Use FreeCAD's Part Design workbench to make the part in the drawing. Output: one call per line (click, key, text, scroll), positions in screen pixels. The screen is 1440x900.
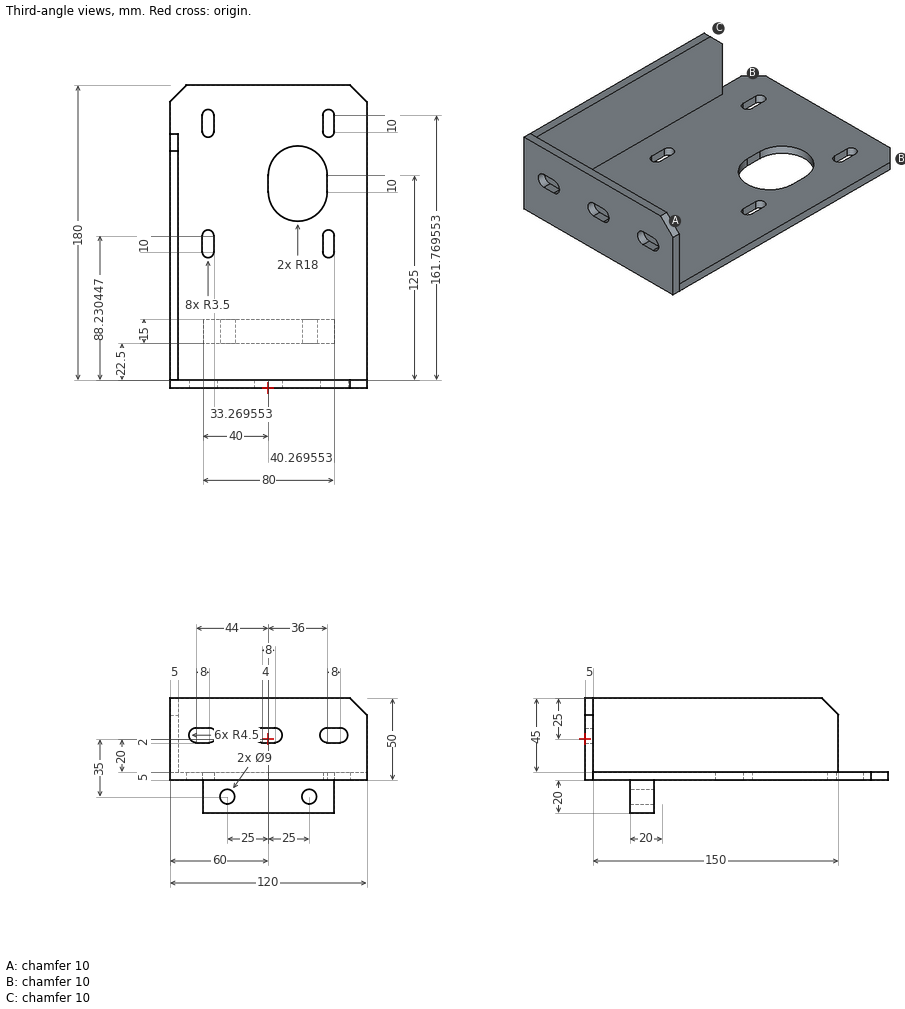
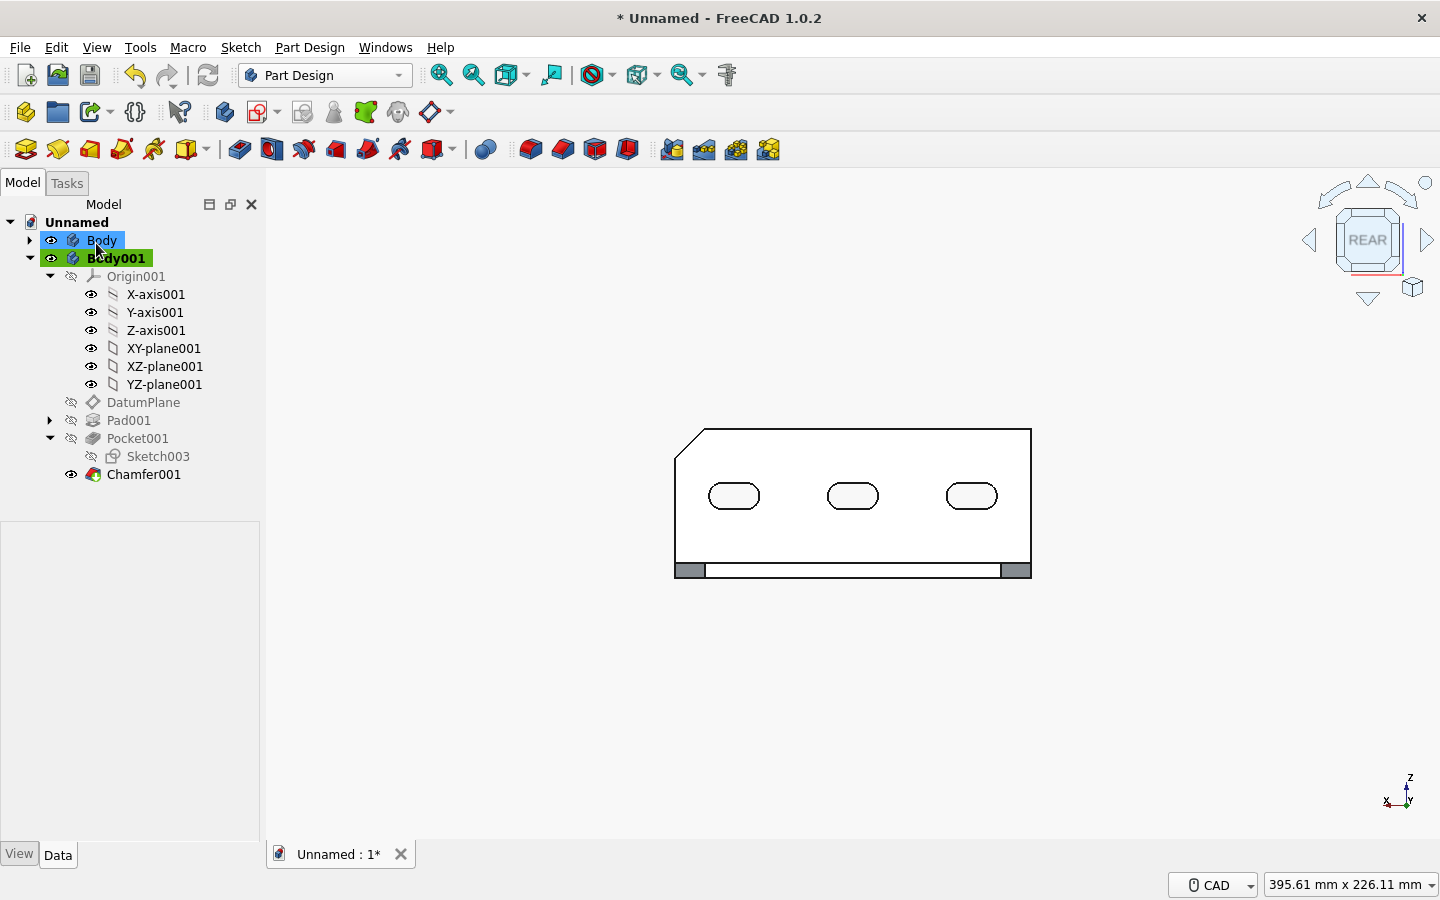
click(442, 76)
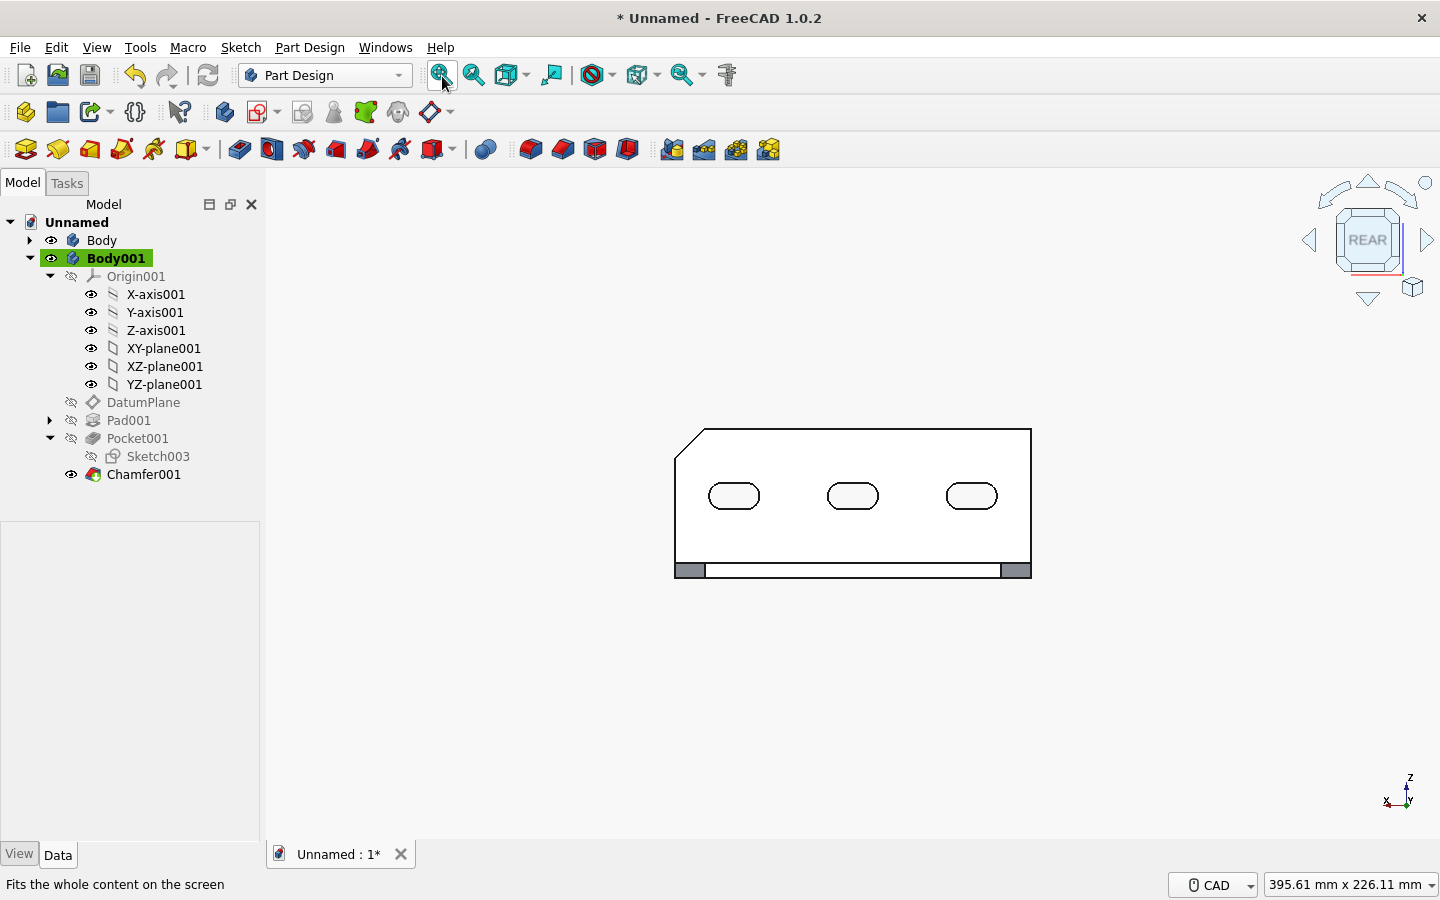
key(5)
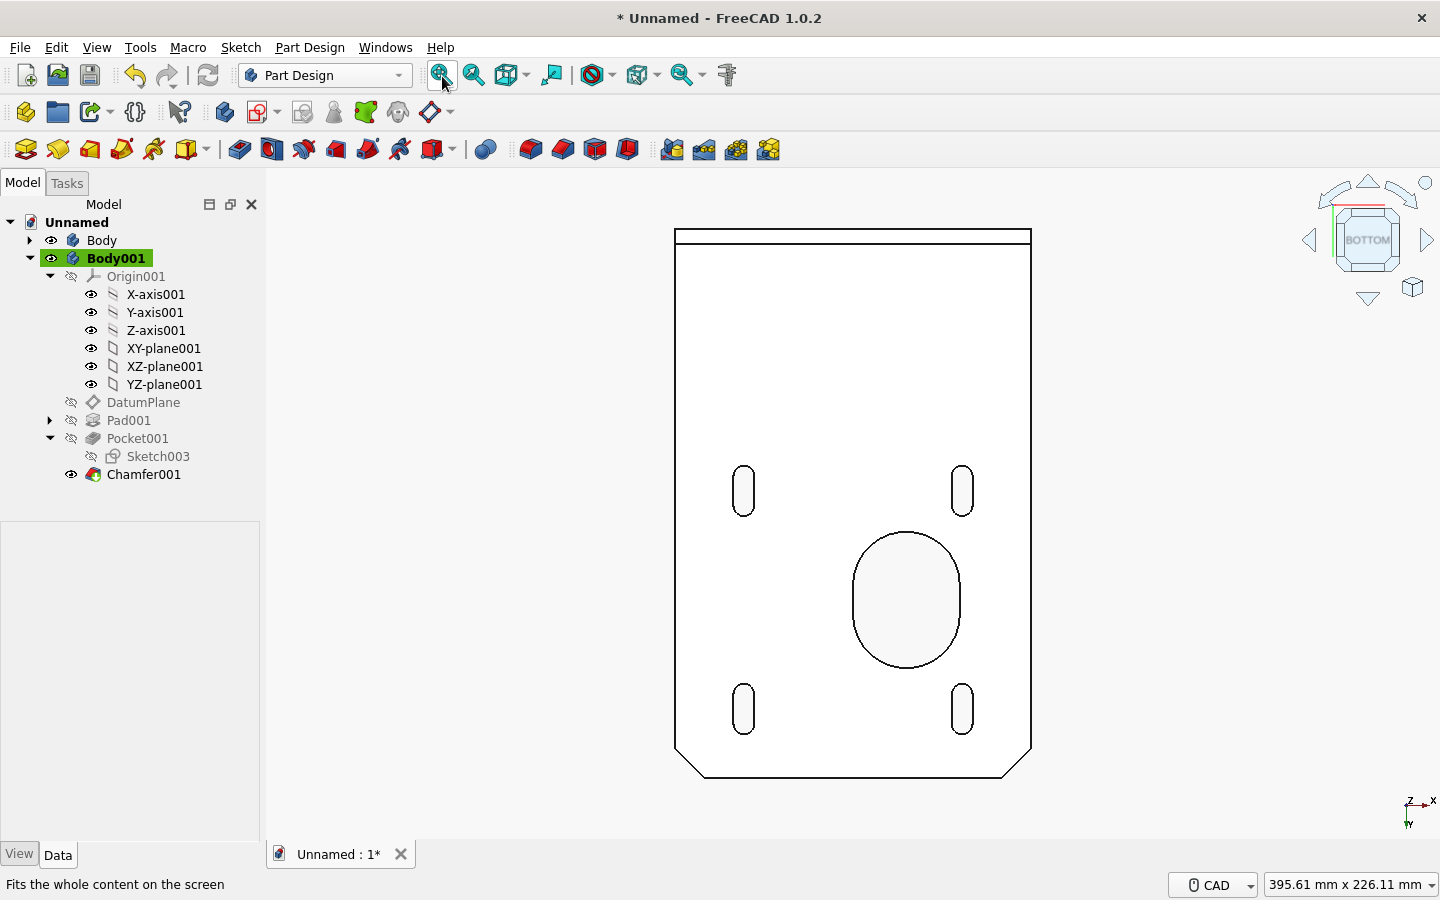
click(904, 357)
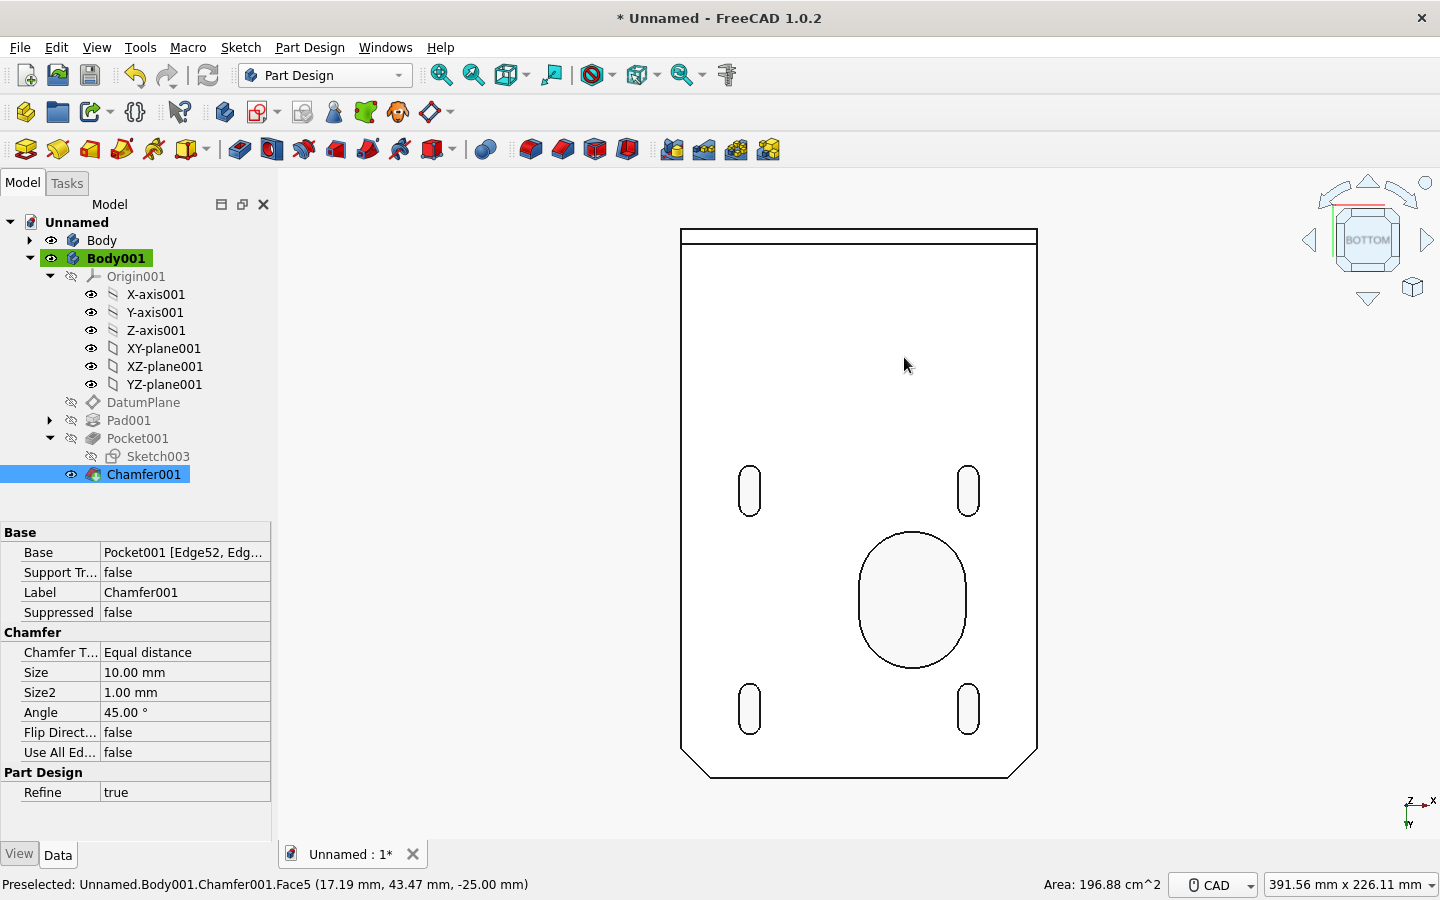
click(258, 112)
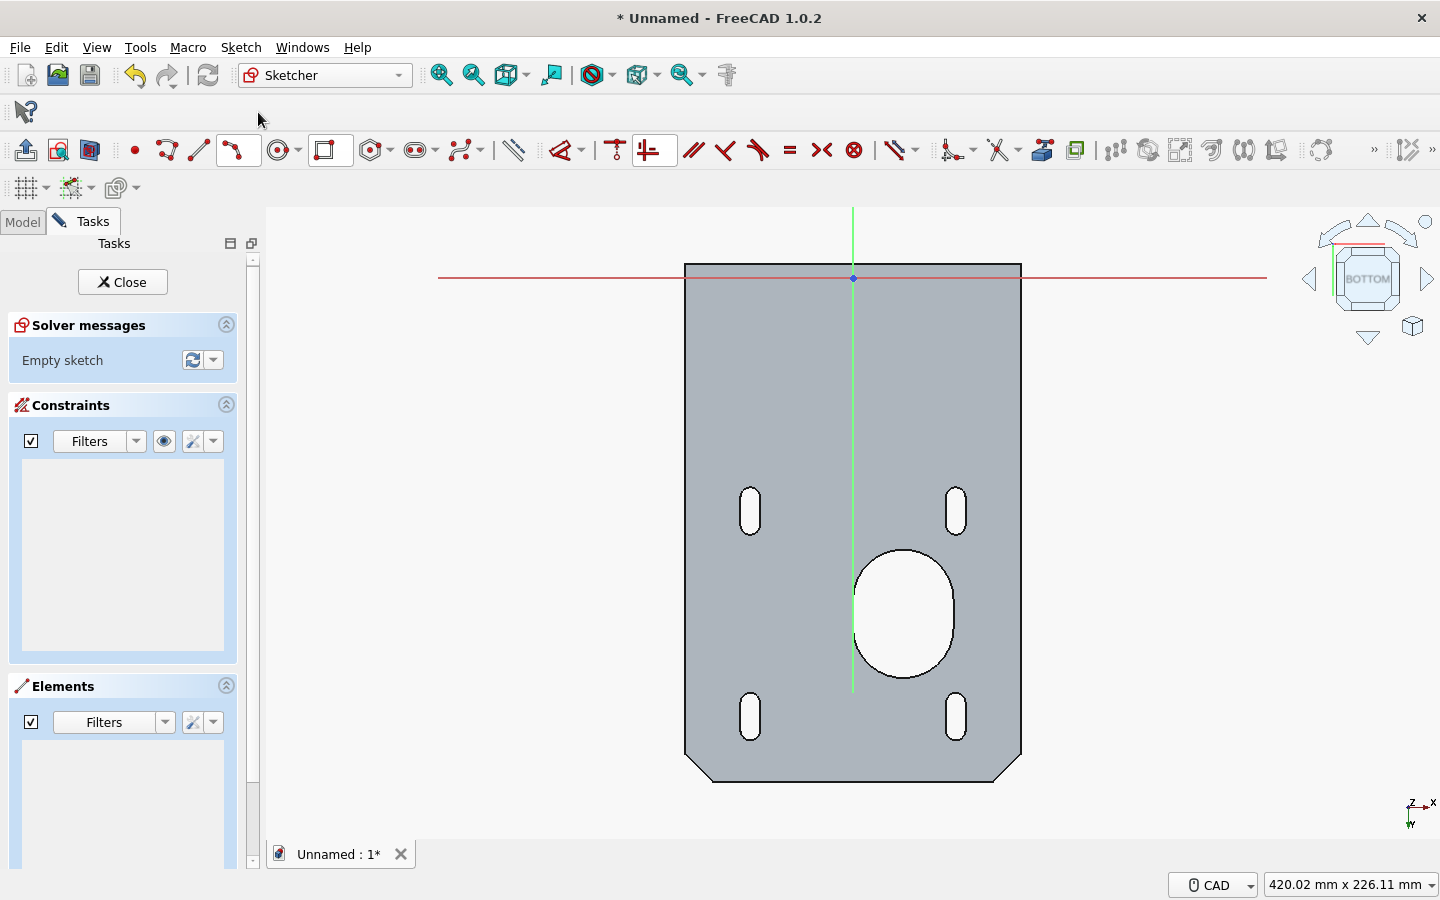
scroll(883, 248, up, 6)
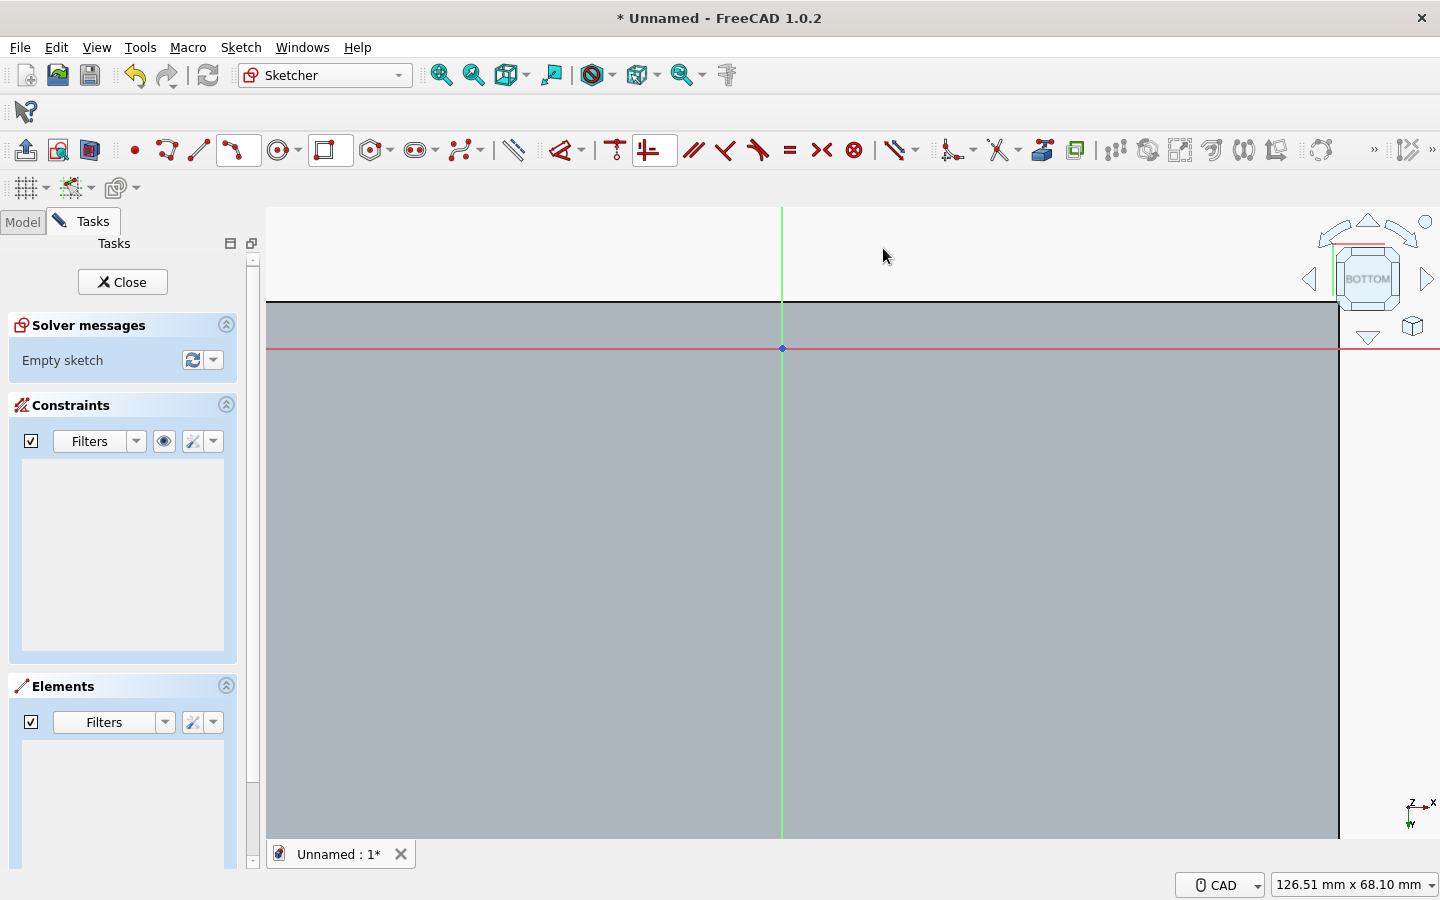
key(g)
key(r)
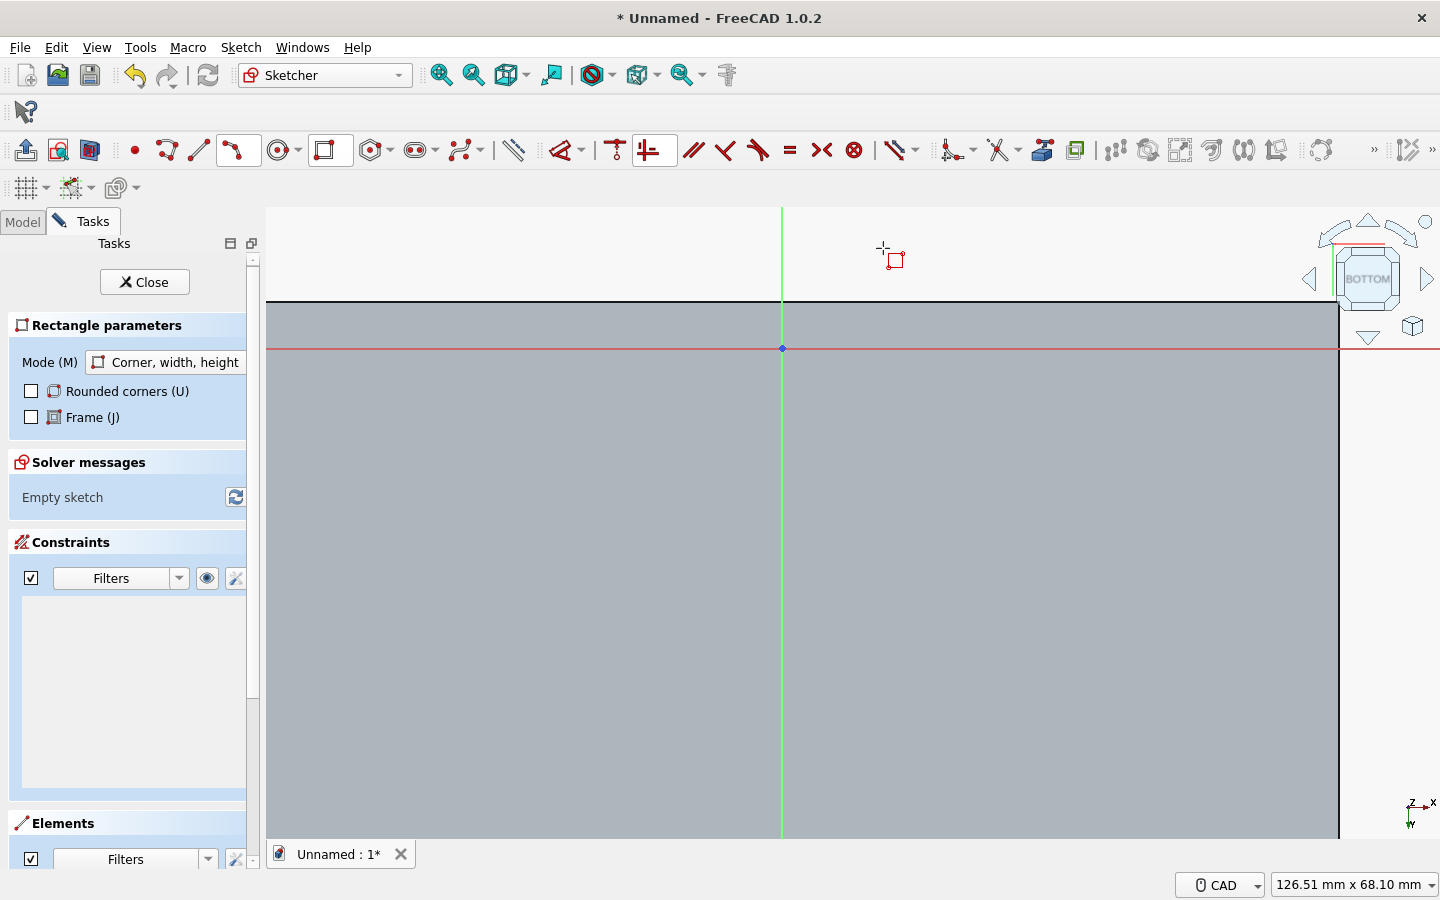
click(411, 558)
click(1153, 697)
key(Escape)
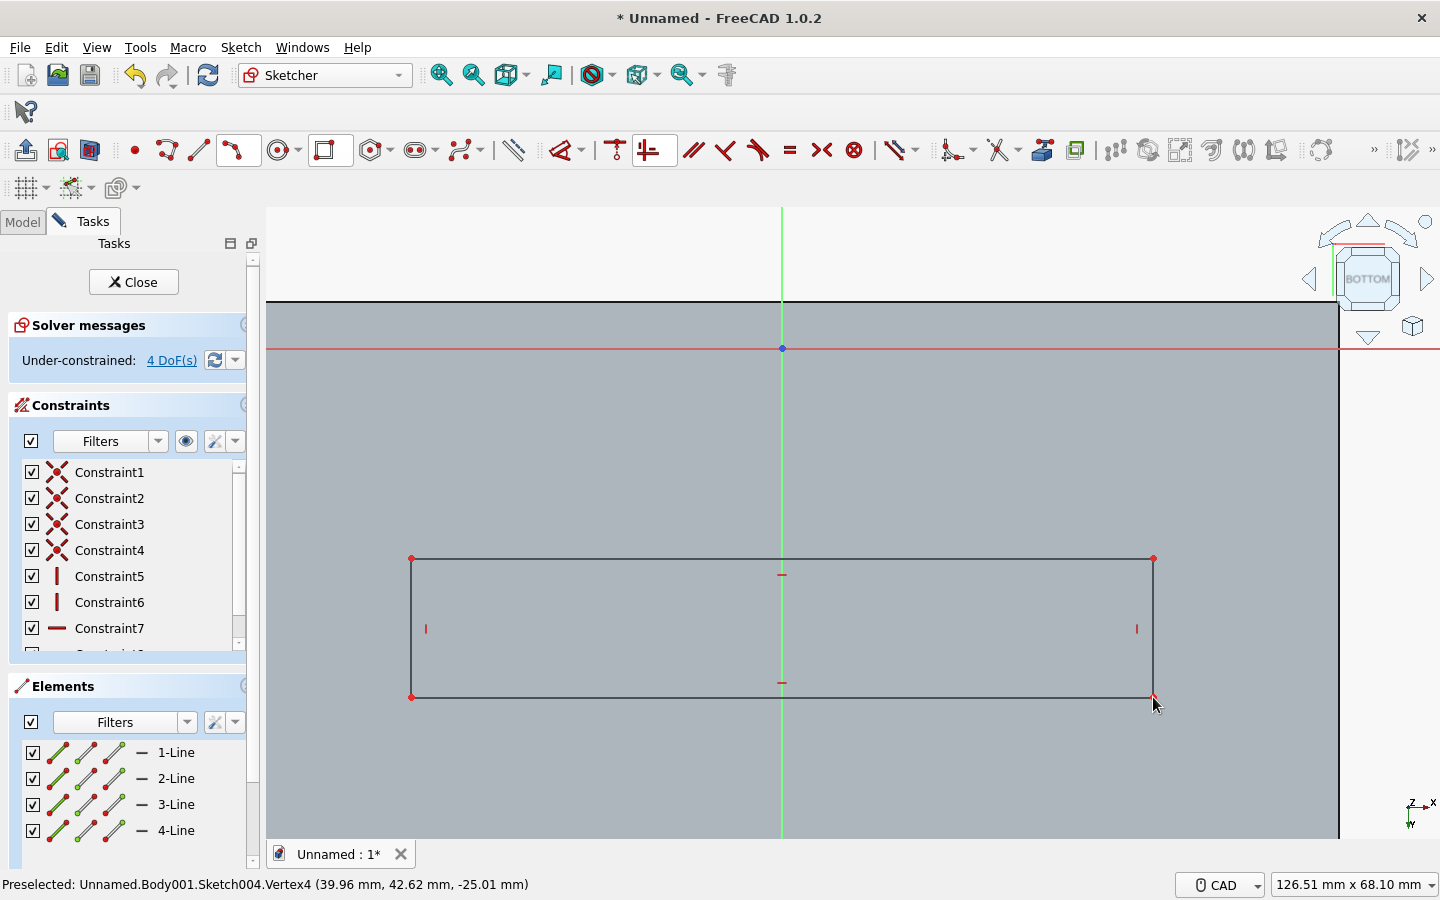
key(d)